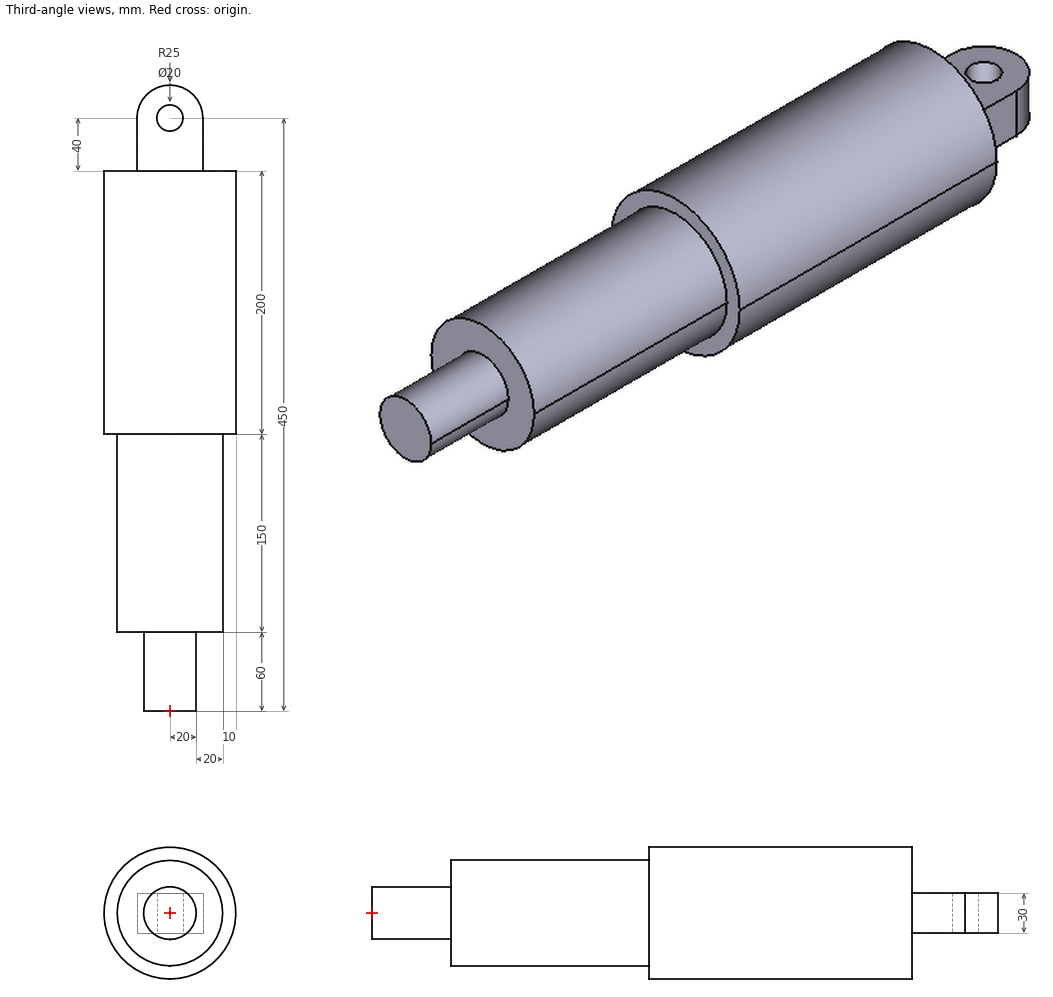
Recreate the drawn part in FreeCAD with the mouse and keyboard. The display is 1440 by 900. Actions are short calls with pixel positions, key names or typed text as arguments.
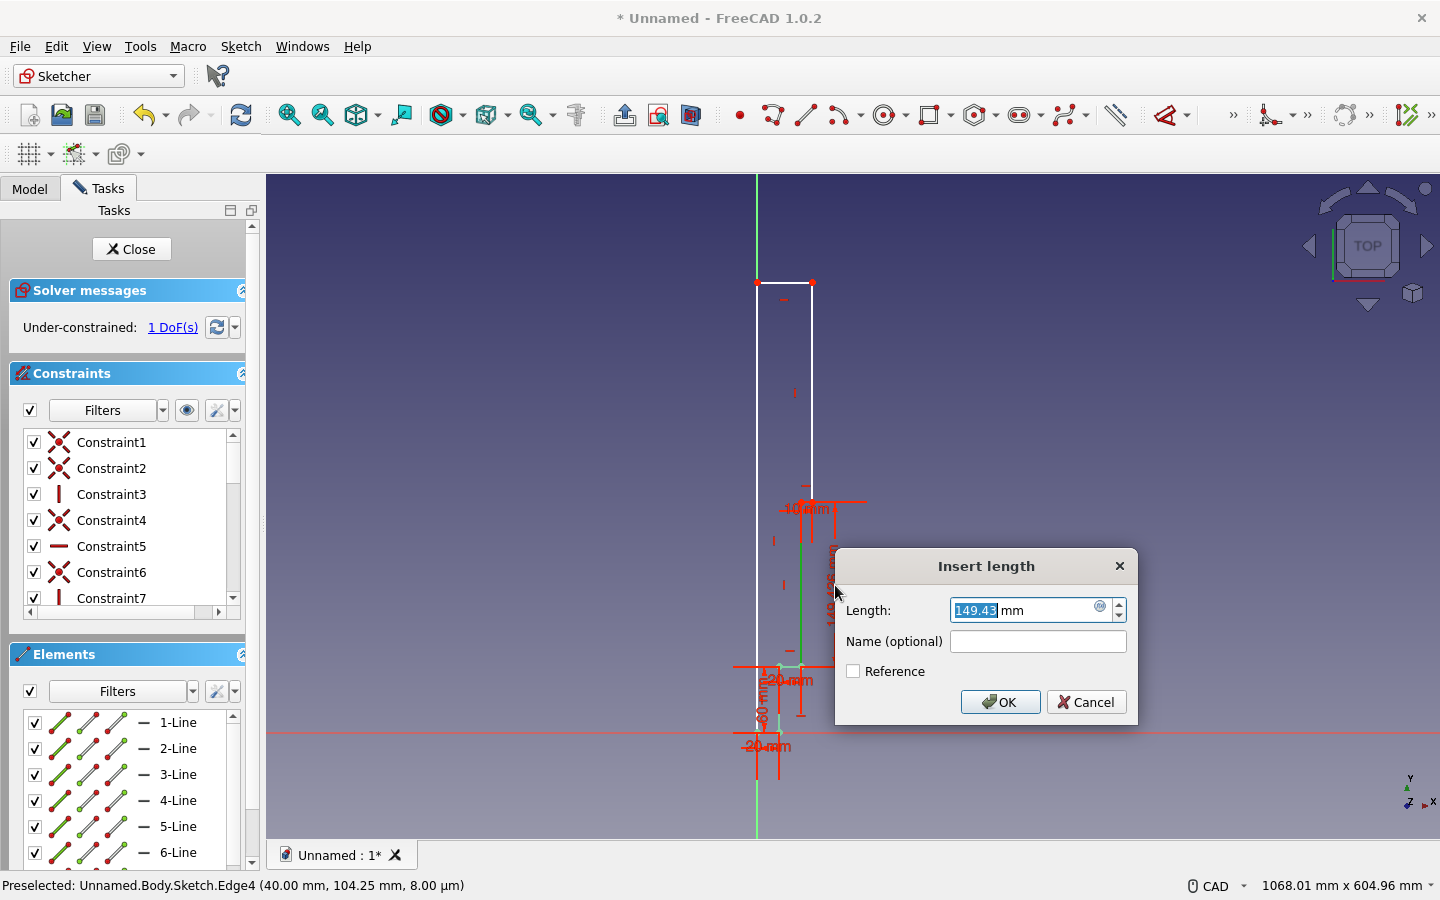
text(150)
key(Return)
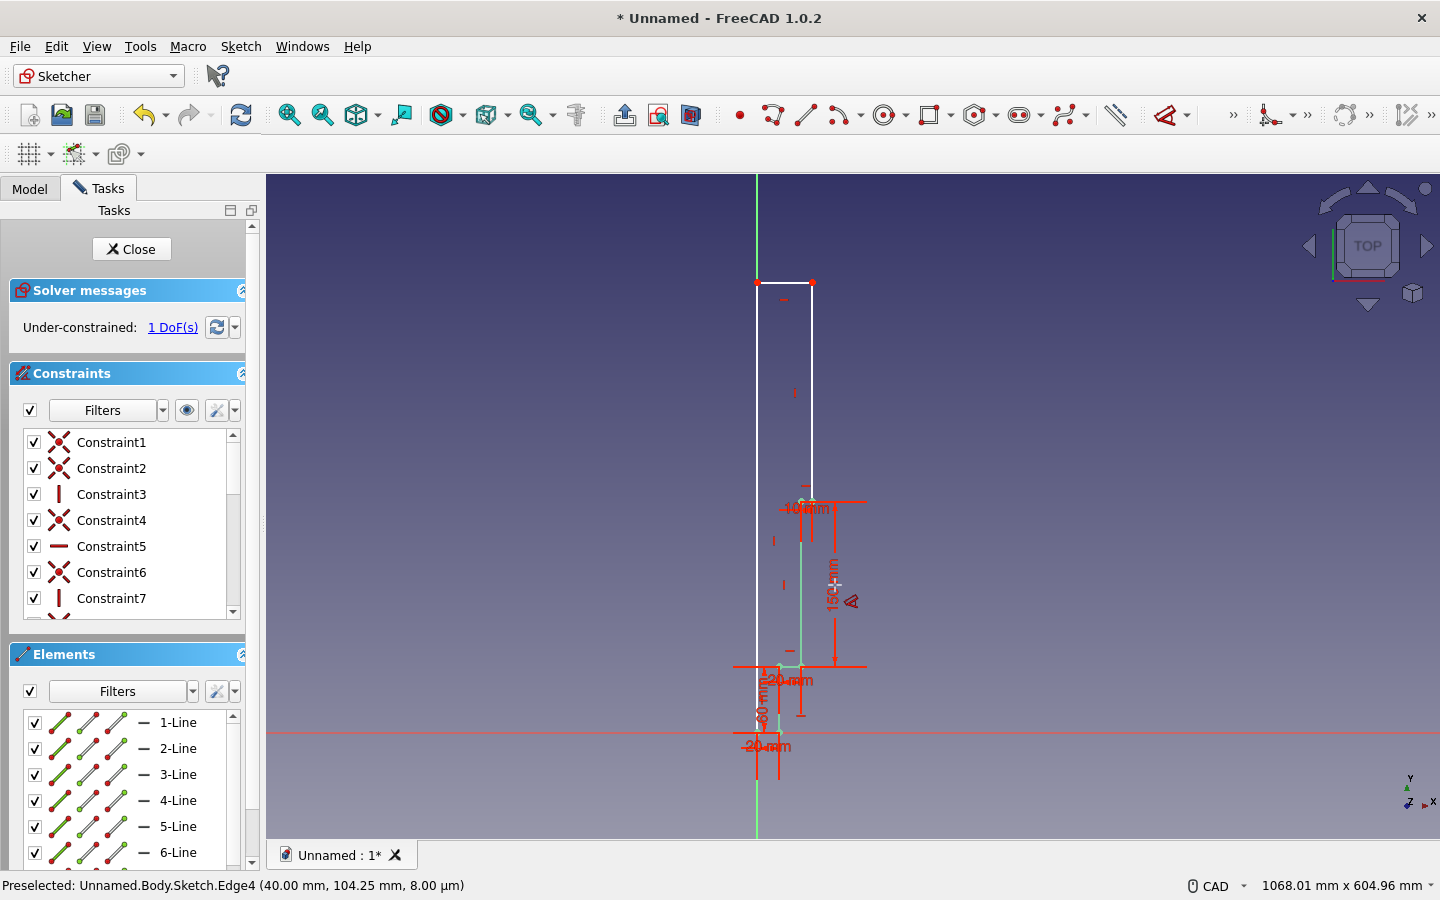
click(812, 436)
click(846, 392)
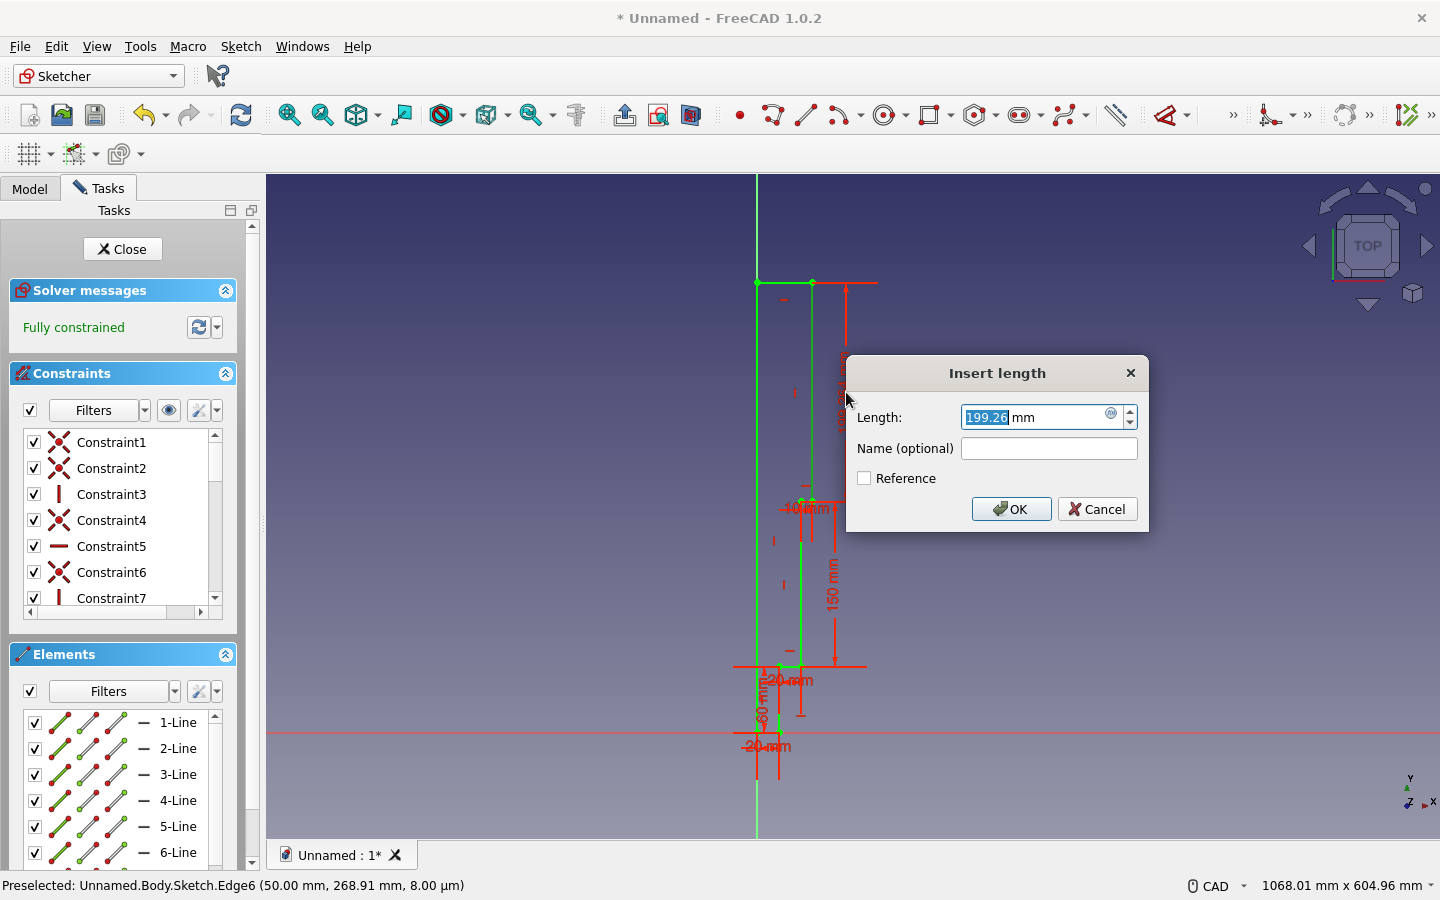
text(200)
key(Return)
key(Escape)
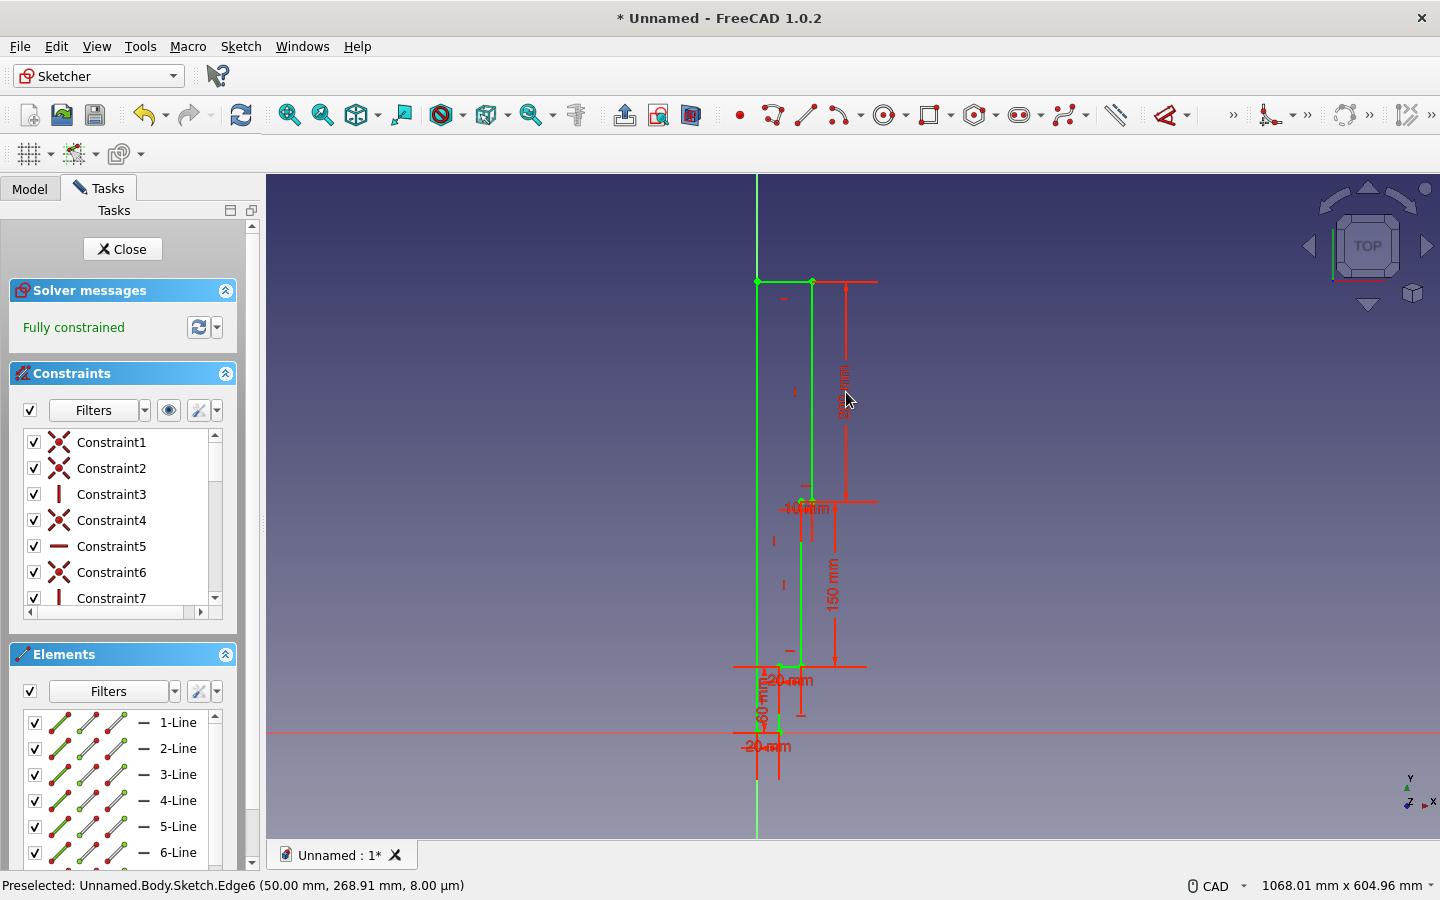
click(123, 249)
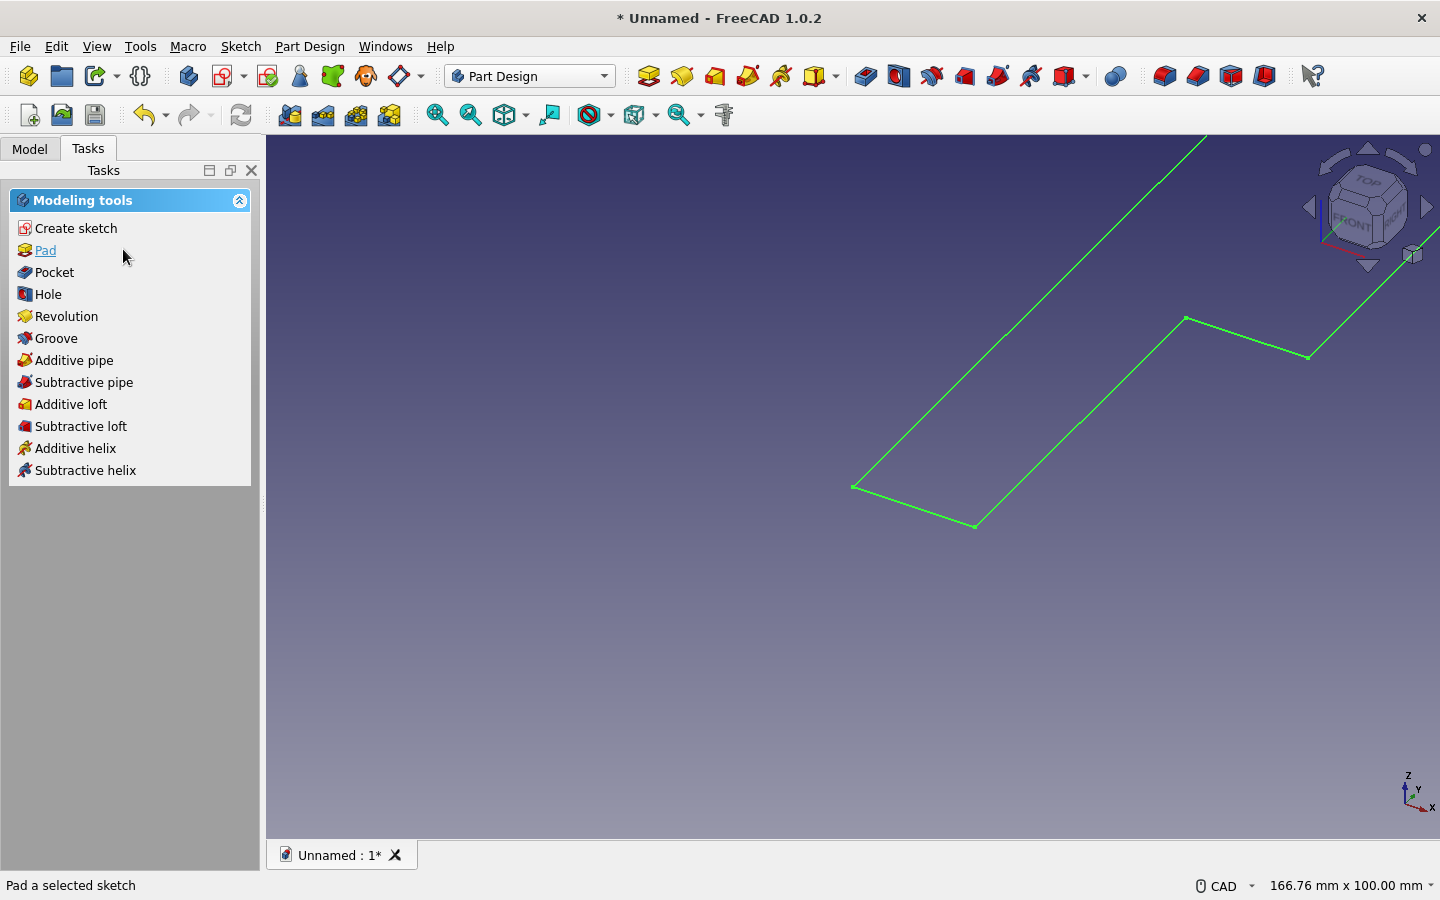
click(682, 76)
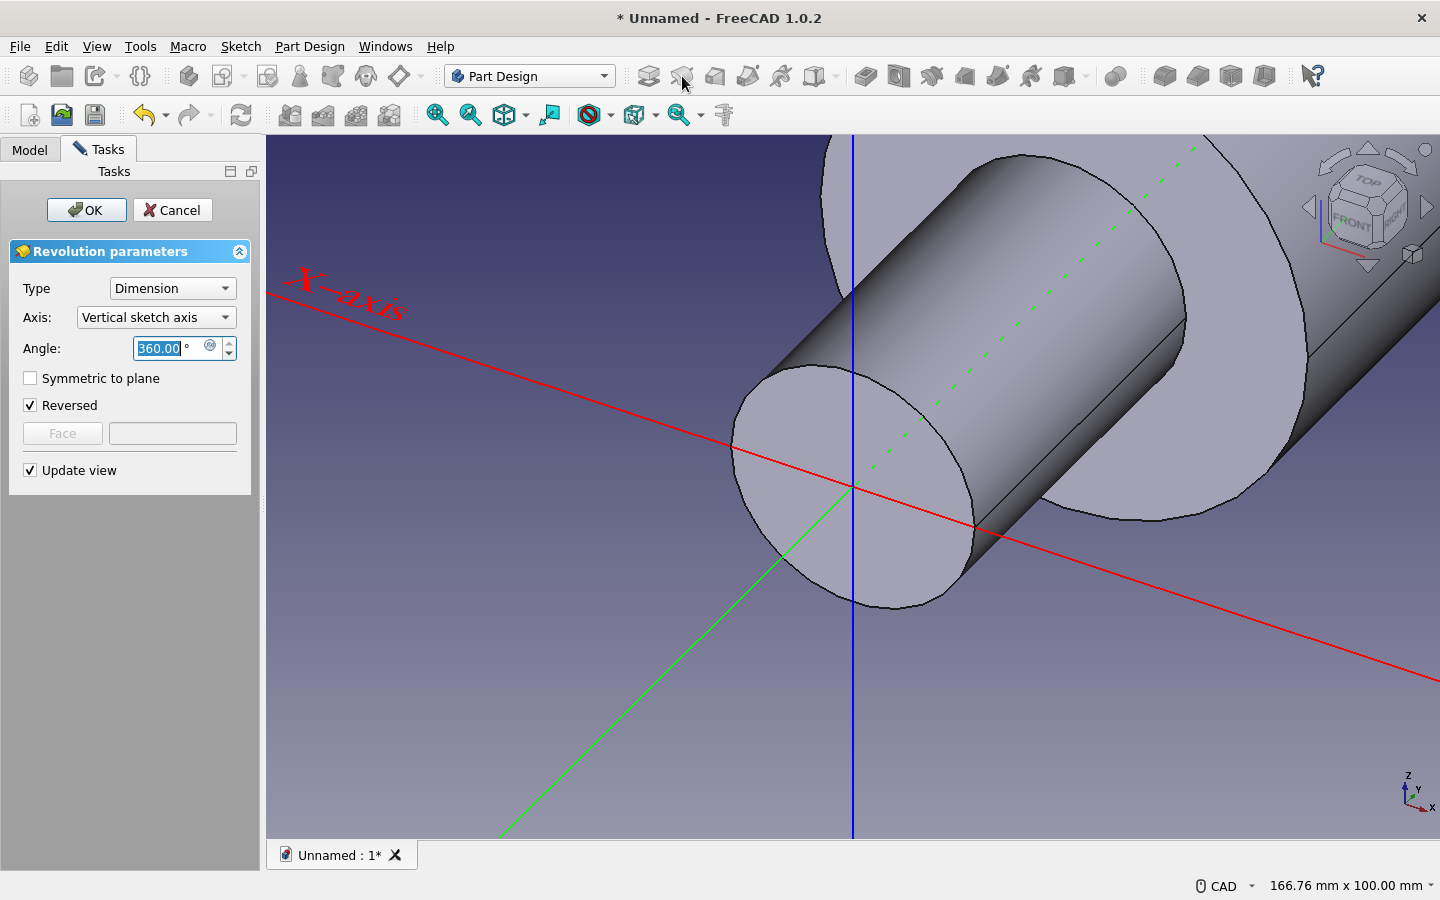
click(87, 210)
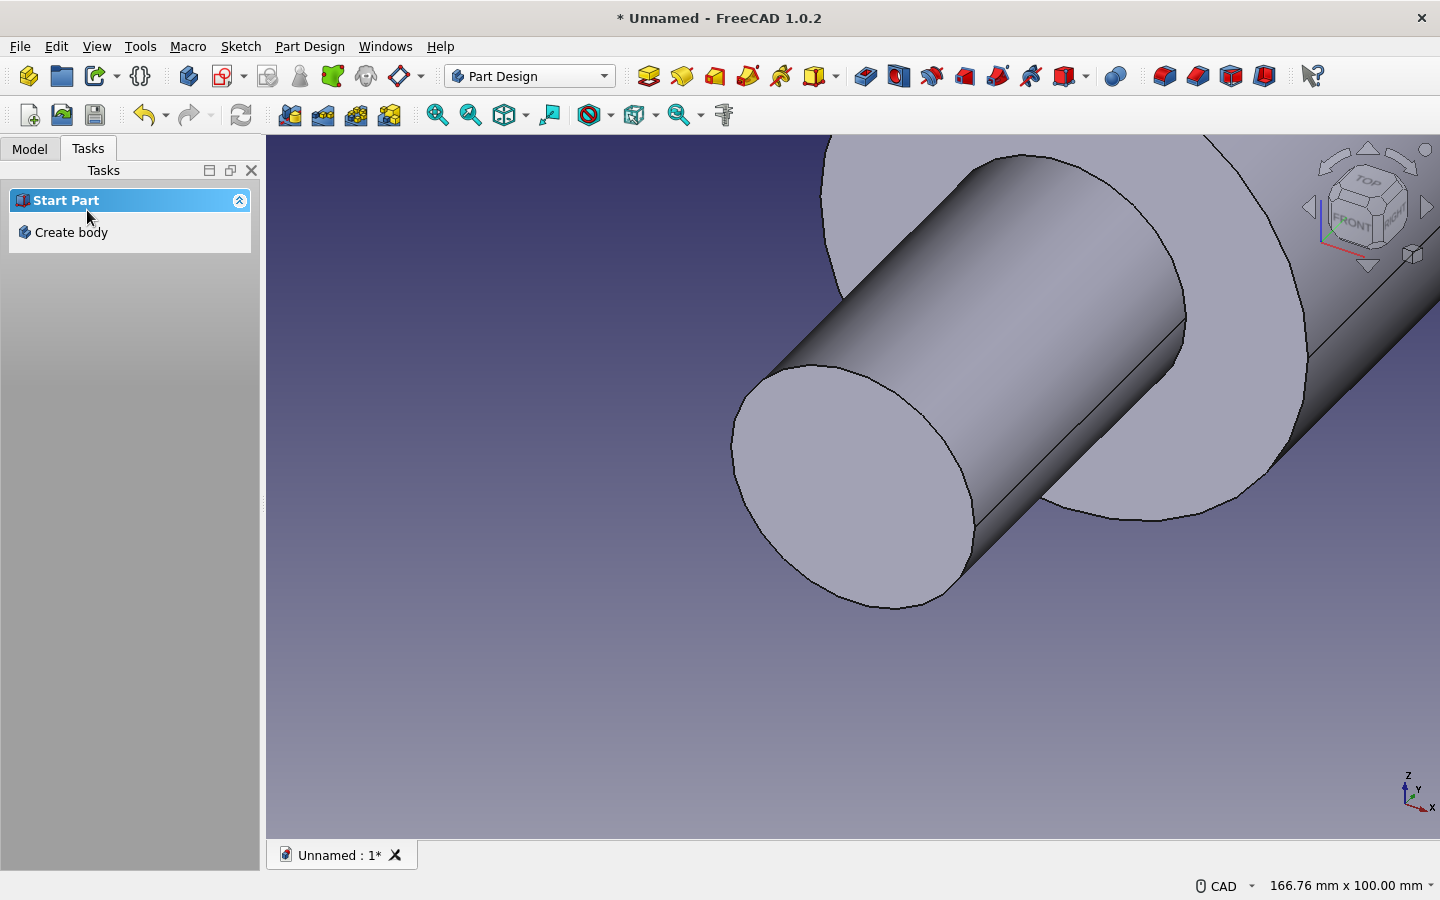
click(438, 116)